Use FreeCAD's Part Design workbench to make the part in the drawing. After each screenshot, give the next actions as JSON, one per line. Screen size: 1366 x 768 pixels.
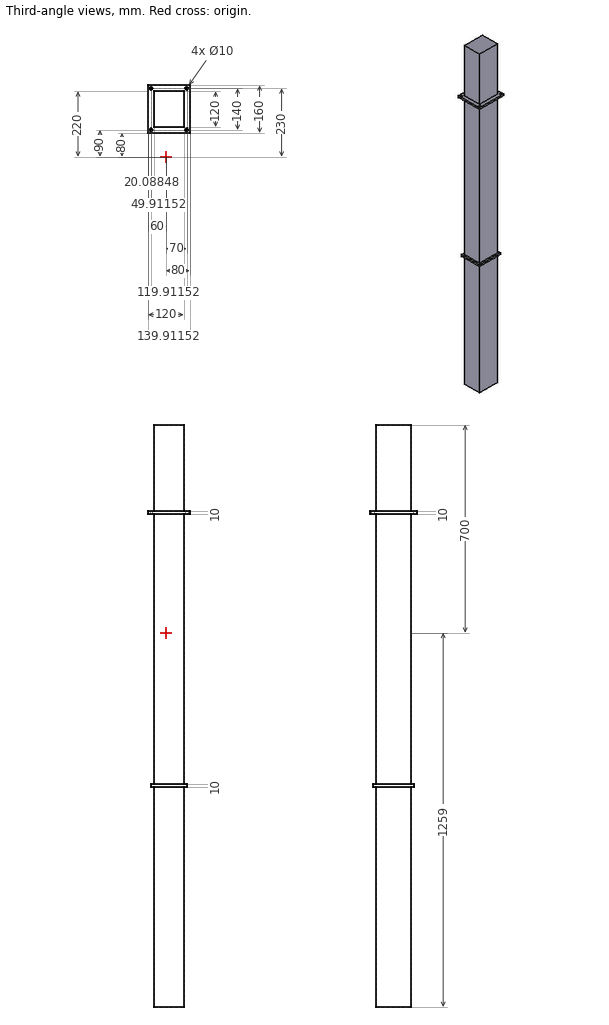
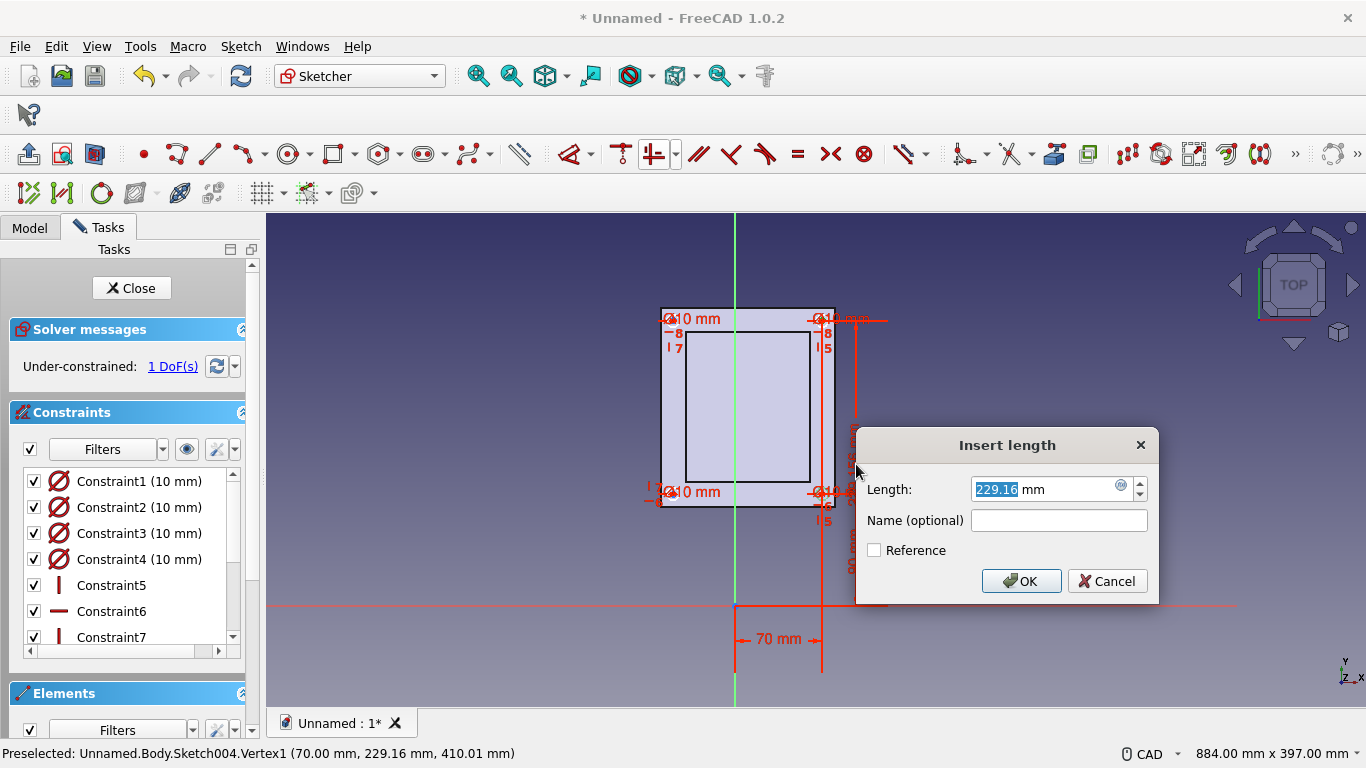
{"action": "type", "text": "230"}
{"action": "key", "text": "Return"}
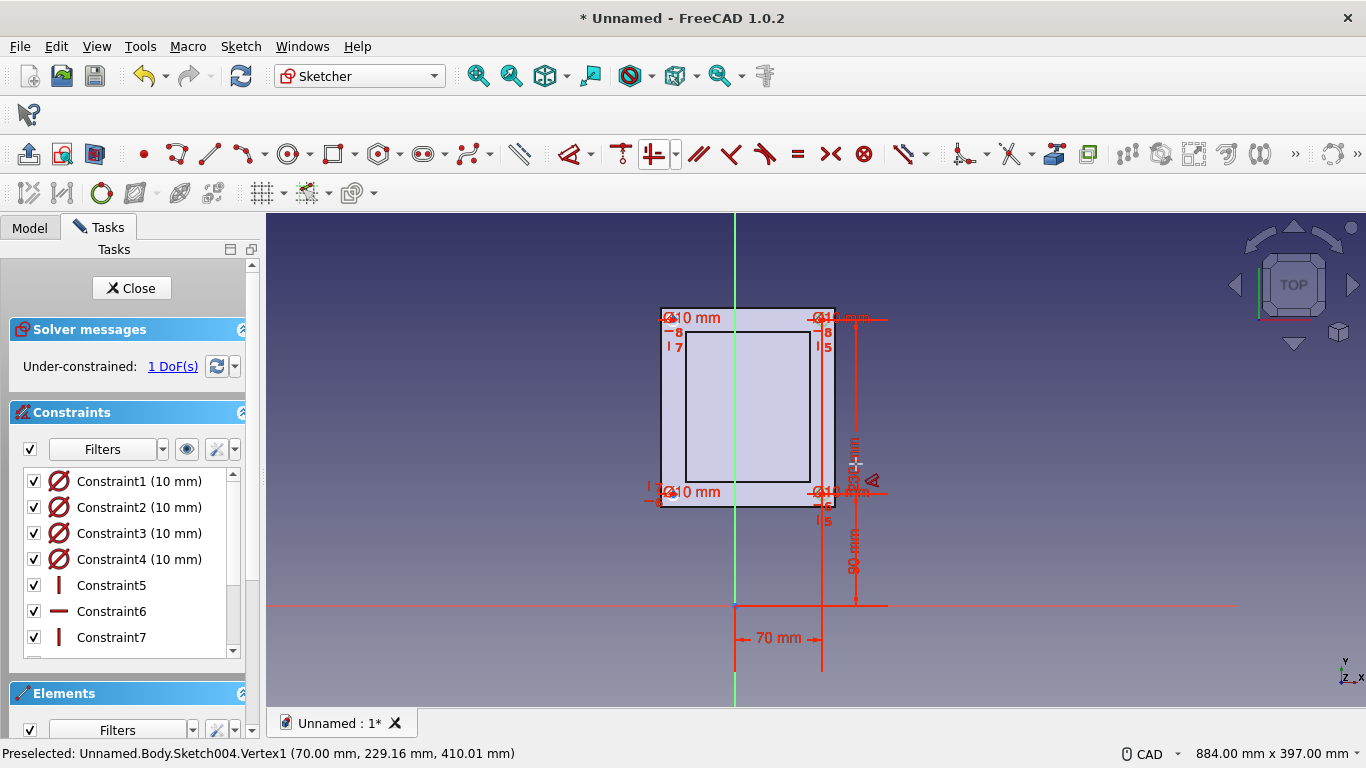
{"action": "left_click", "coordinate": [673, 494]}
{"action": "left_click", "coordinate": [704, 640]}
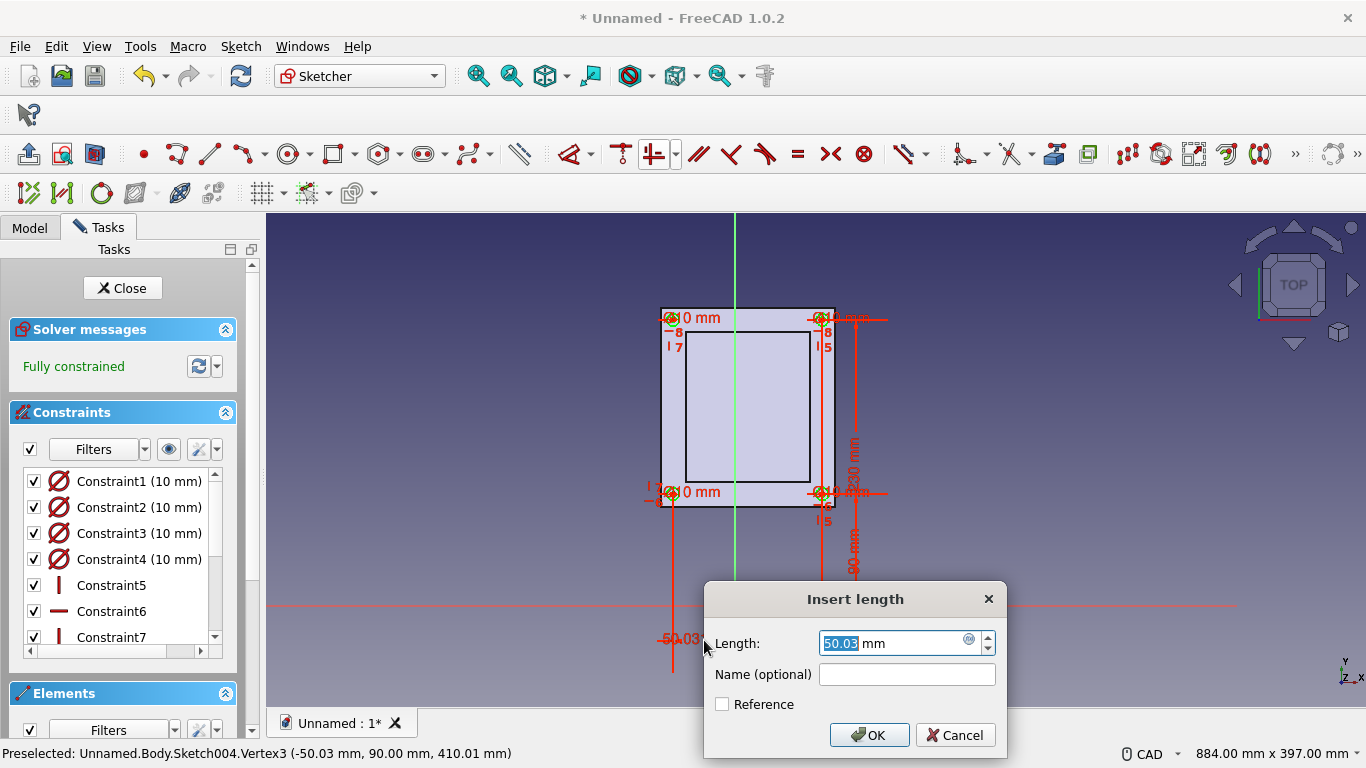
{"action": "type", "text": "49.91152"}
{"action": "key", "text": "Return"}
{"action": "key", "text": "Escape"}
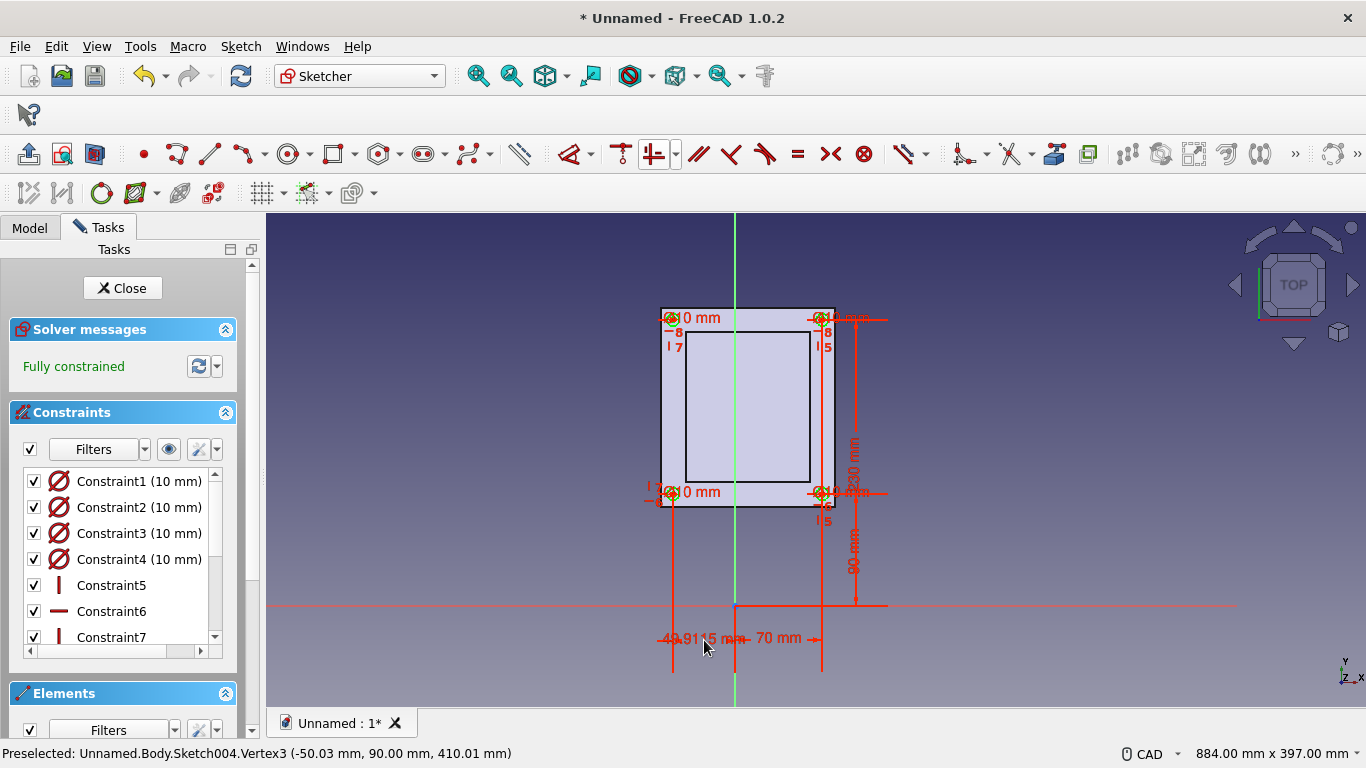
{"action": "left_click", "coordinate": [123, 288]}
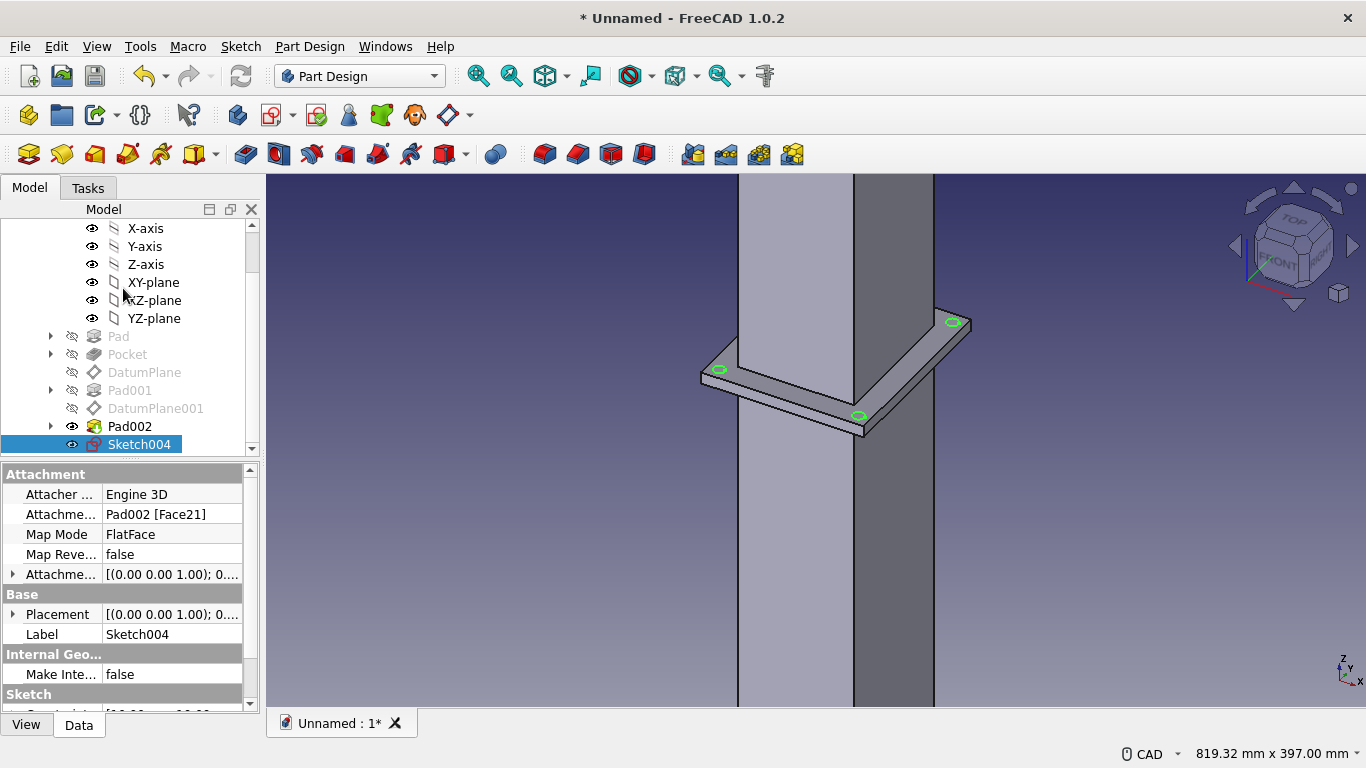
{"action": "left_click", "coordinate": [246, 154]}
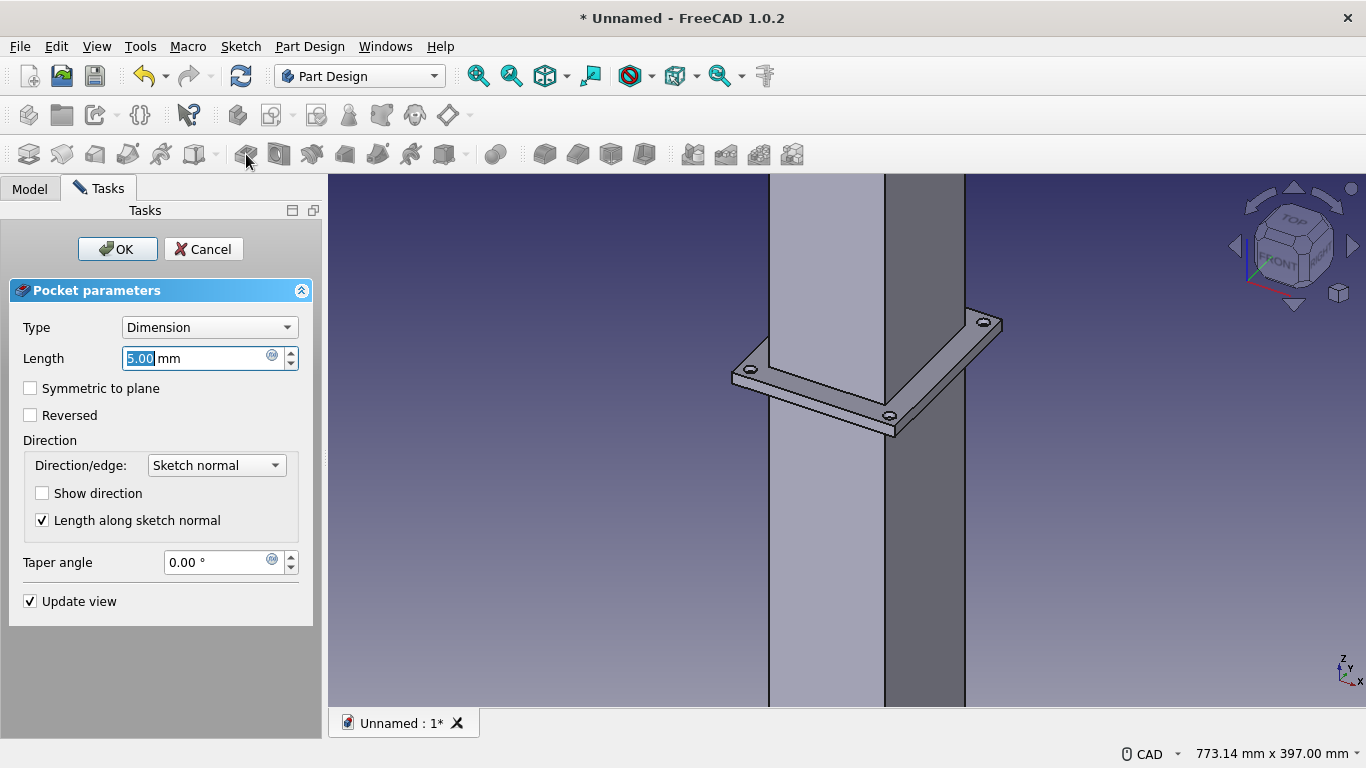
{"action": "type", "text": "10"}
{"action": "key", "text": "Tab"}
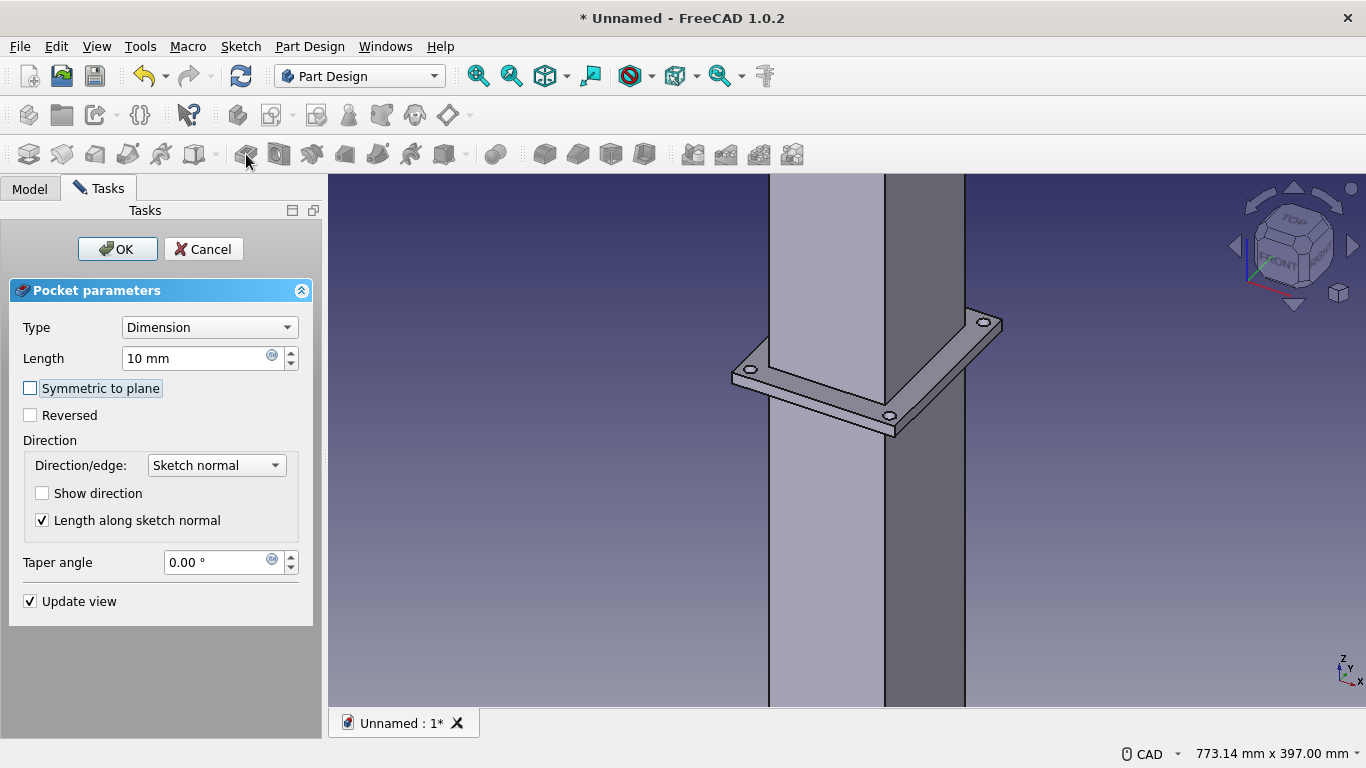
{"action": "left_click", "coordinate": [118, 249]}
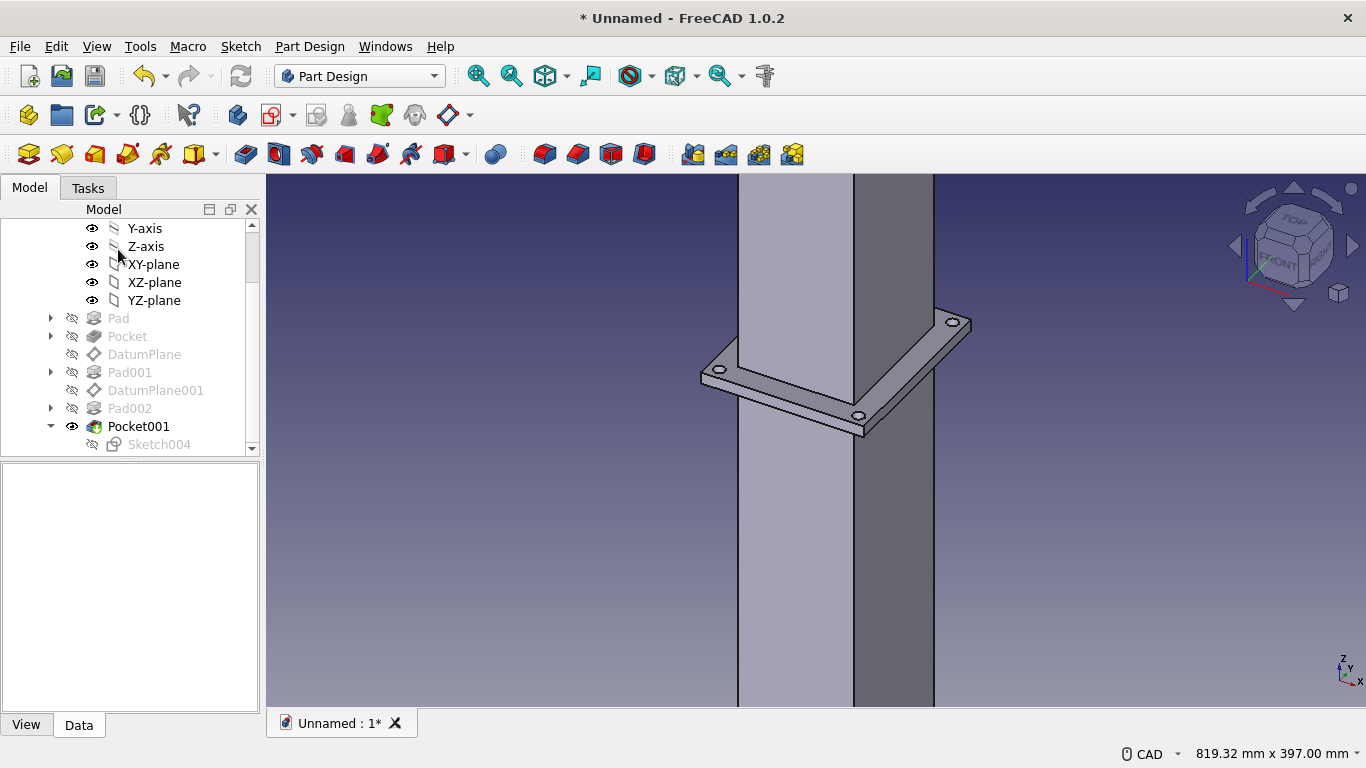
{"action": "key", "text": "0"}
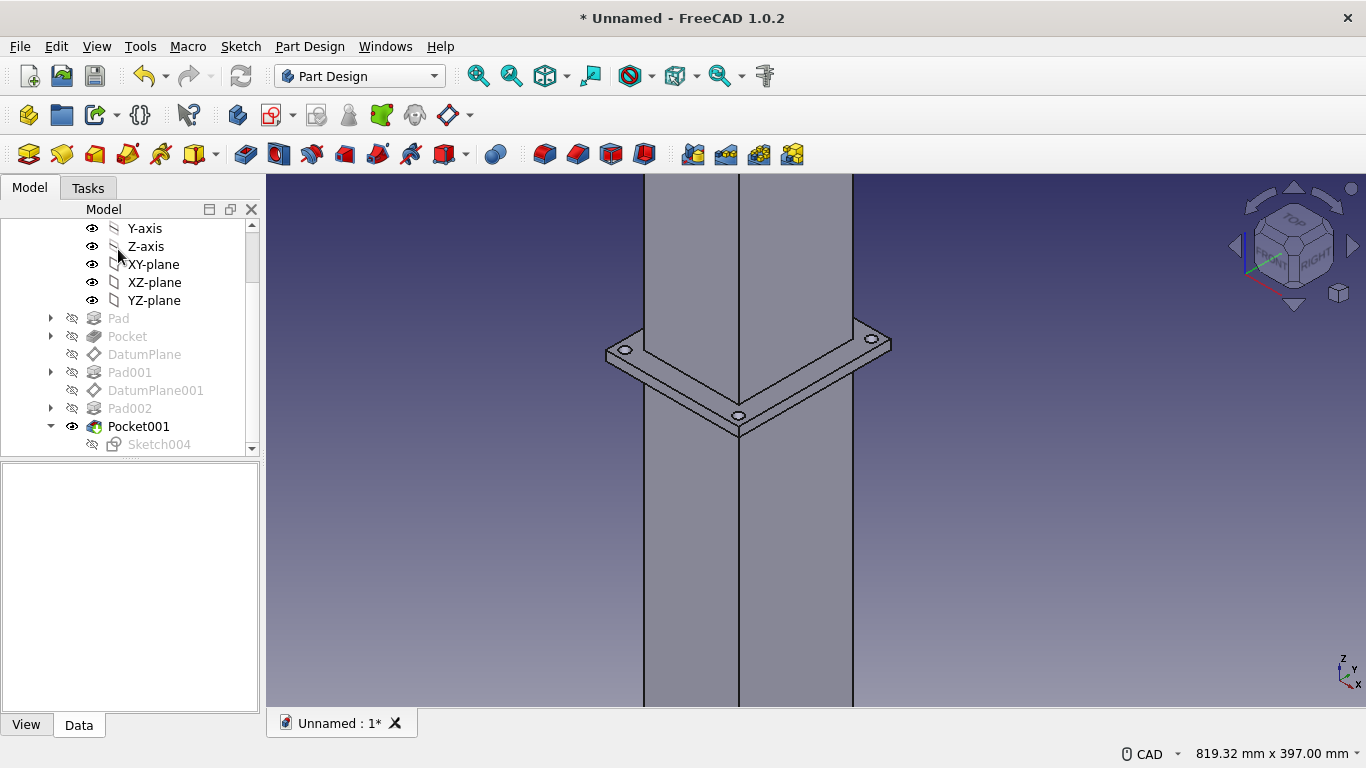
{"action": "left_click", "coordinate": [479, 76]}